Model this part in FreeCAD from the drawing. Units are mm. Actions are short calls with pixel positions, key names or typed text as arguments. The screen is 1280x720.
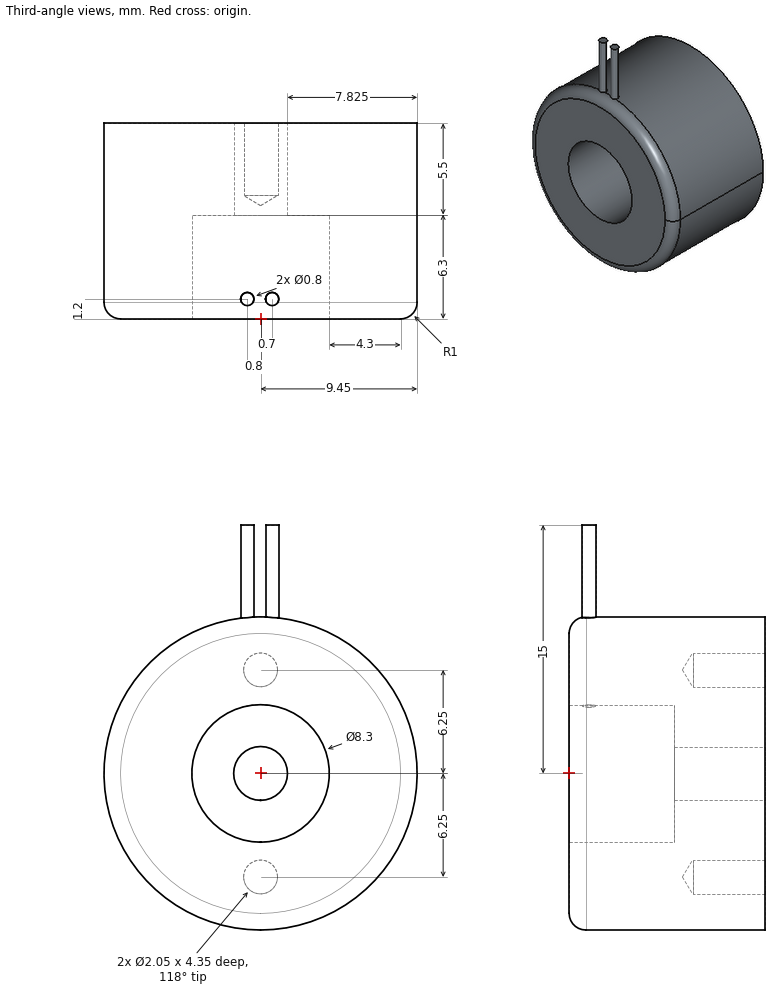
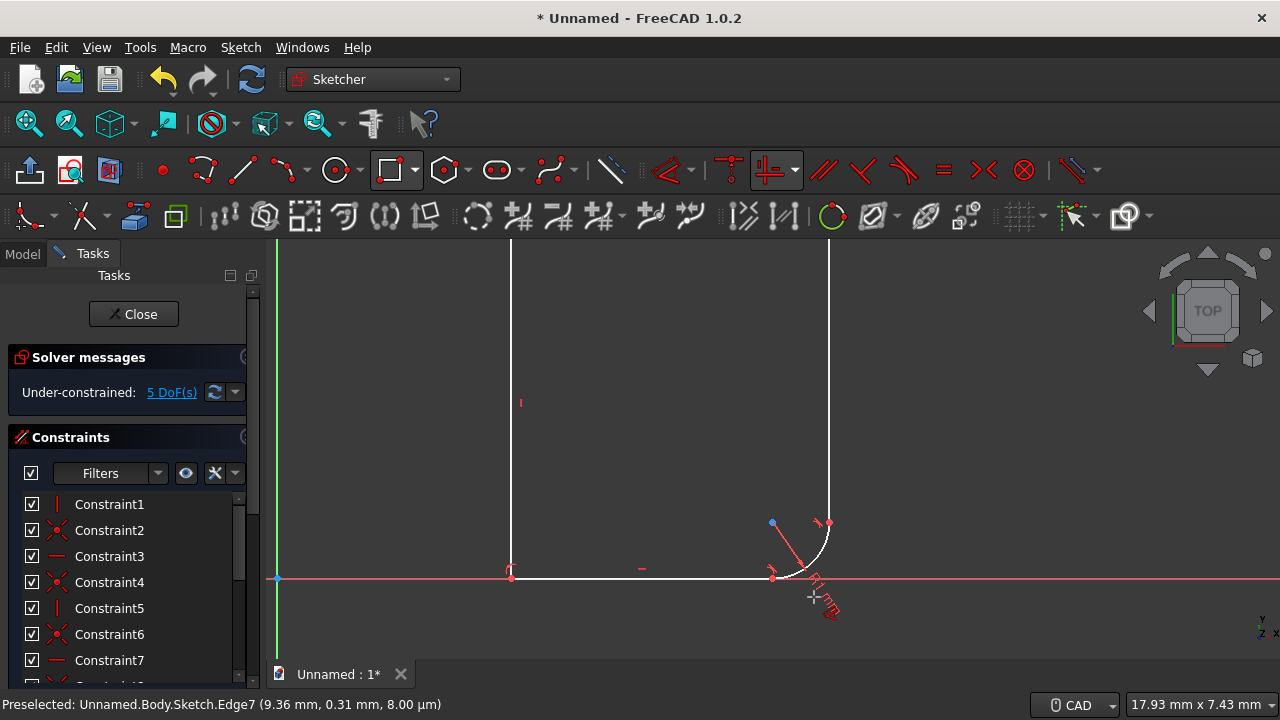
scroll(798, 568, down, 5)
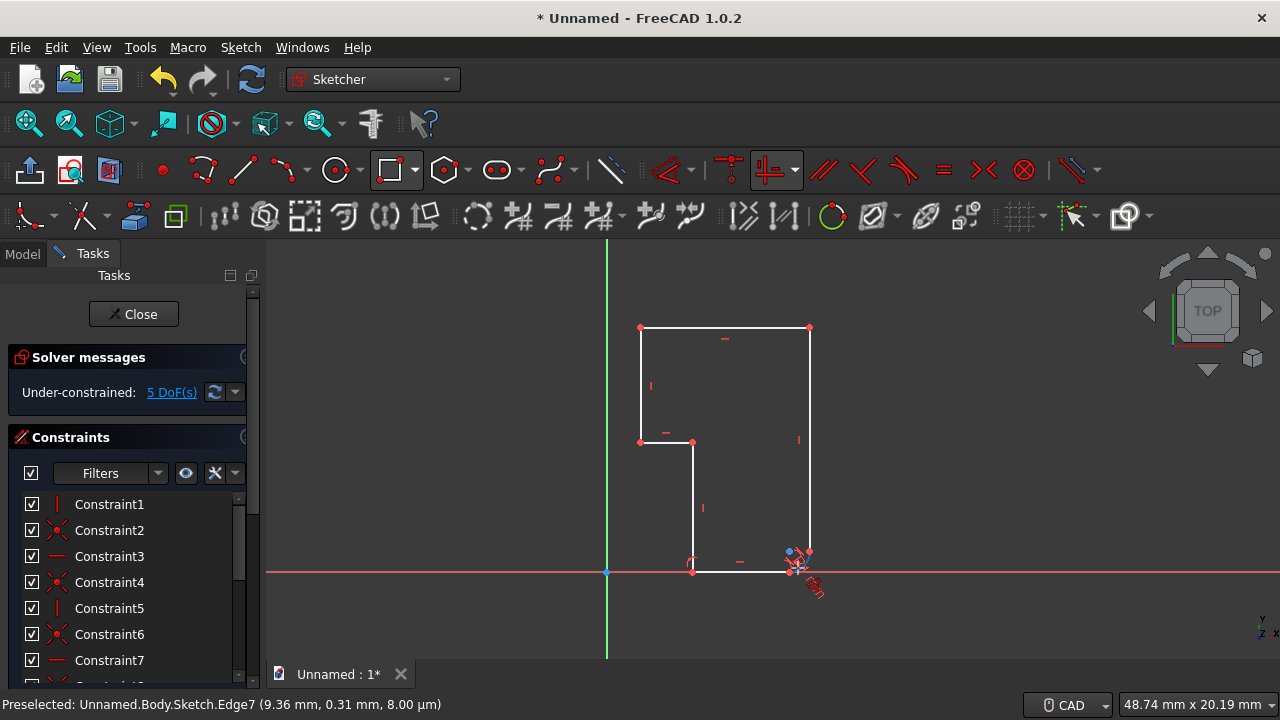
click(641, 362)
click(675, 385)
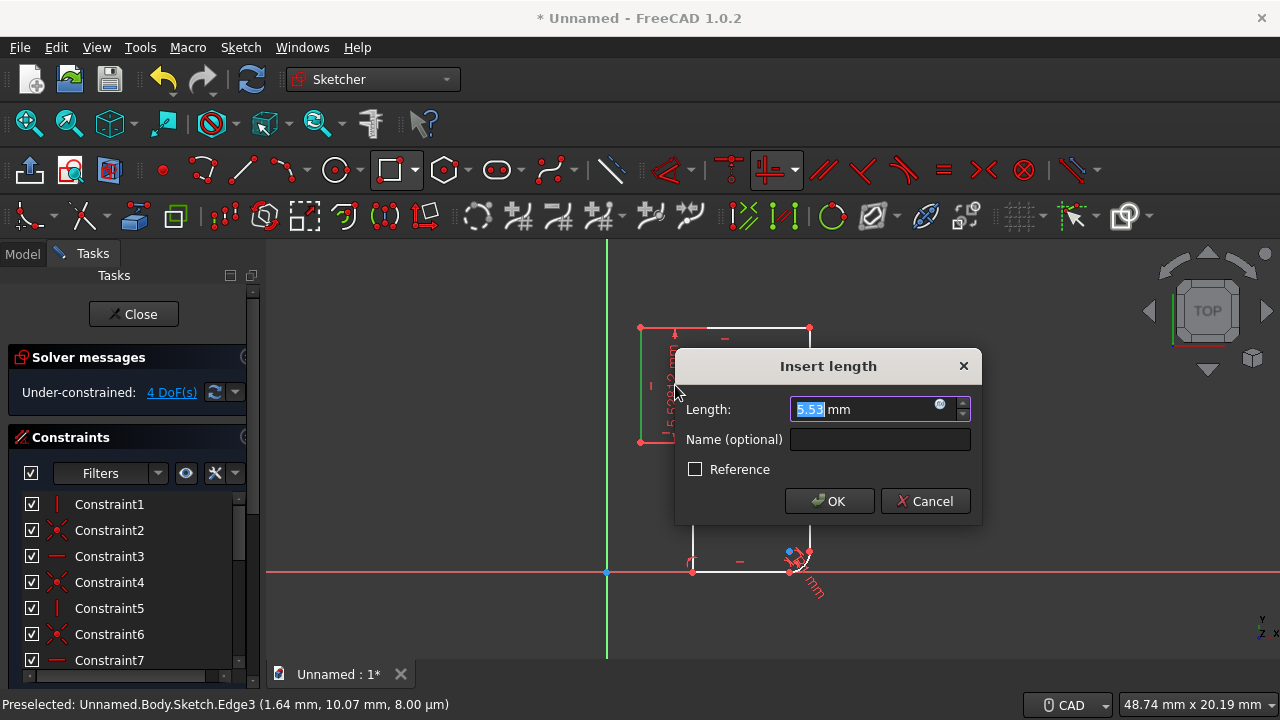
text(5.5)
key(Return)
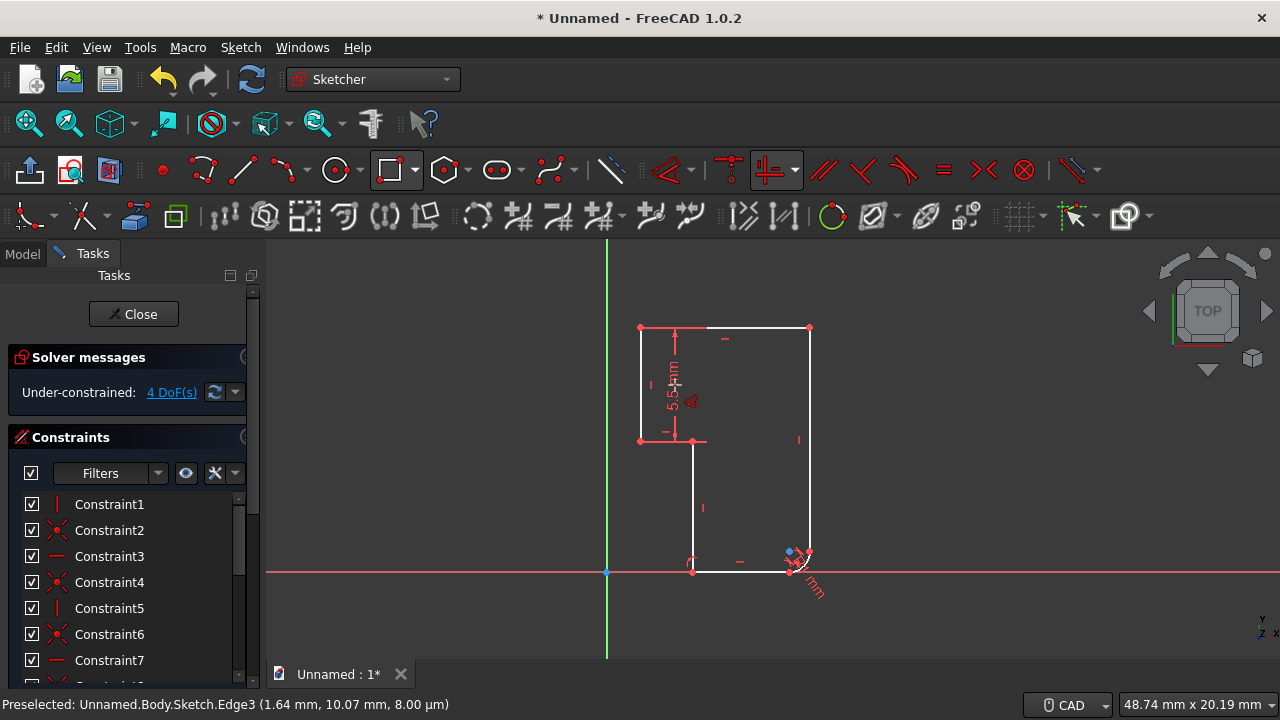
click(693, 481)
click(659, 507)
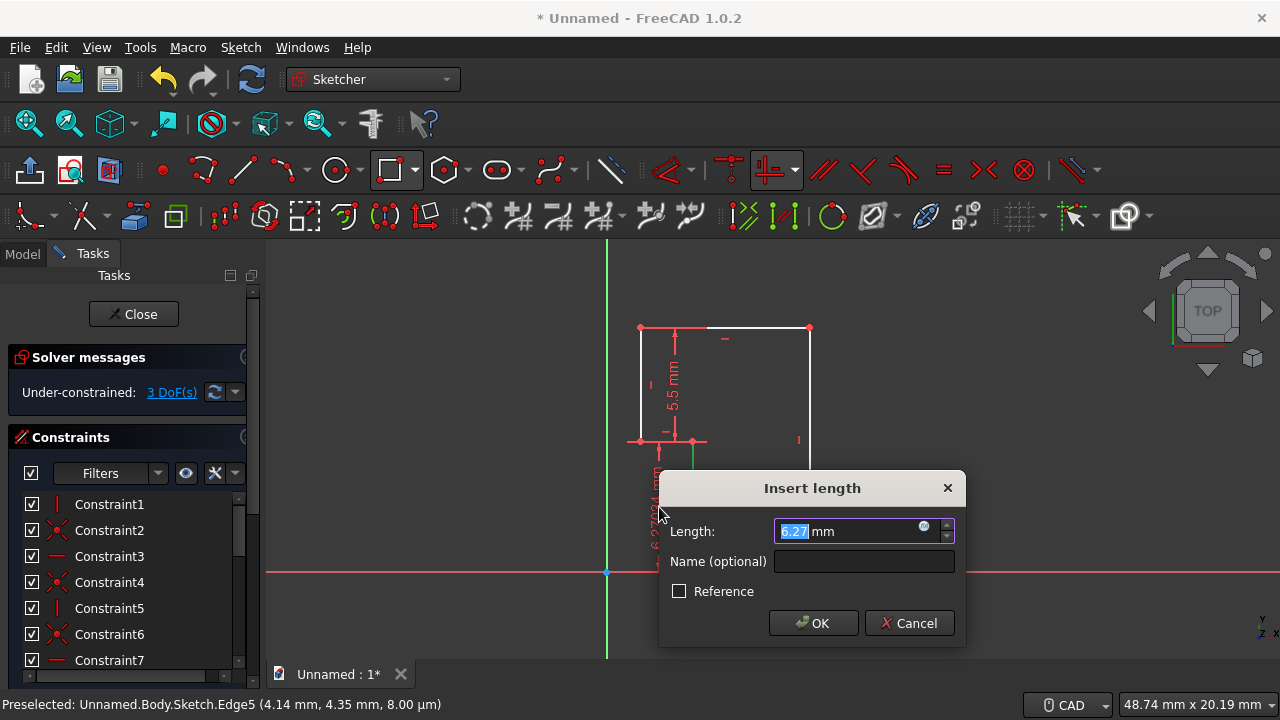
text(6.3)
key(Return)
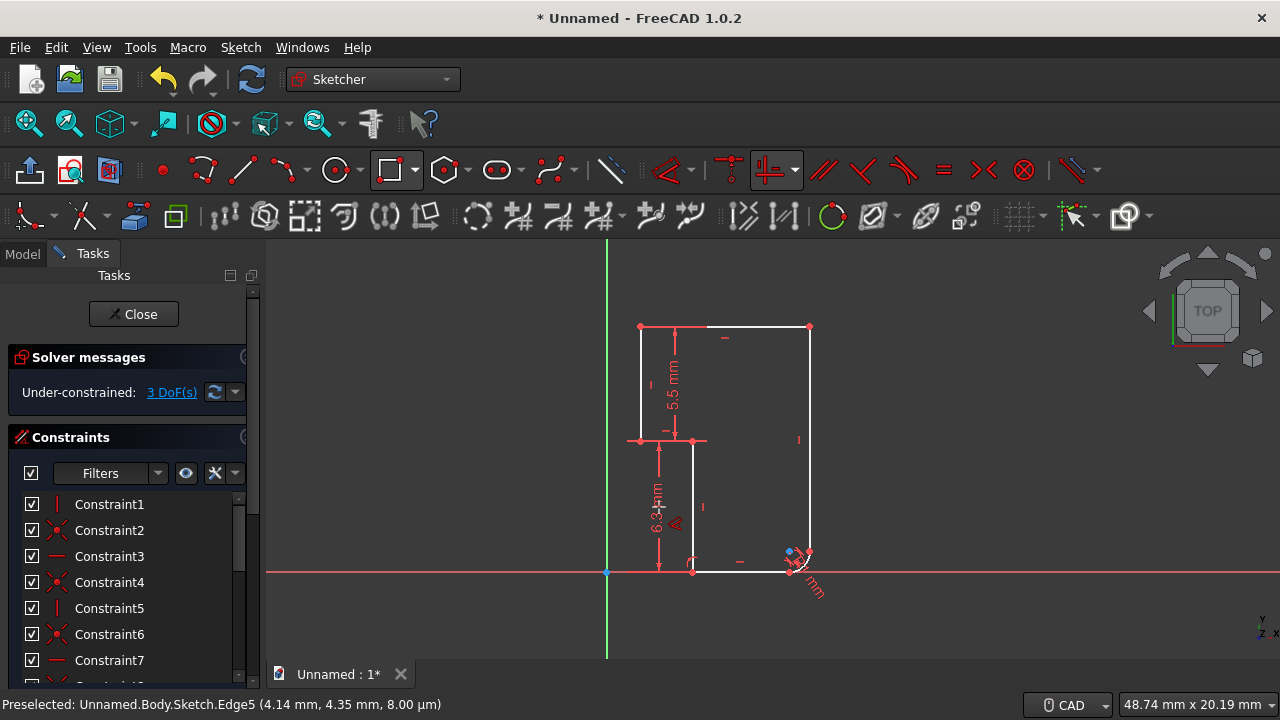
click(722, 572)
click(741, 606)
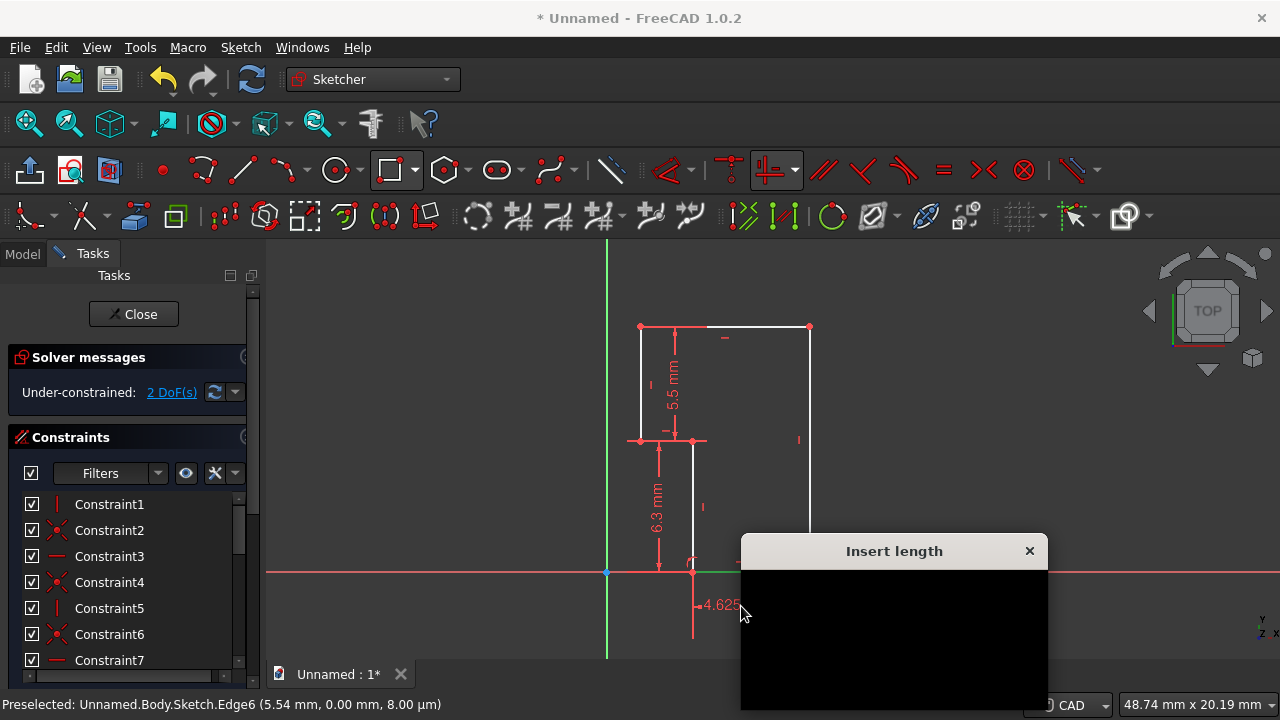
text(4.3)
key(Return)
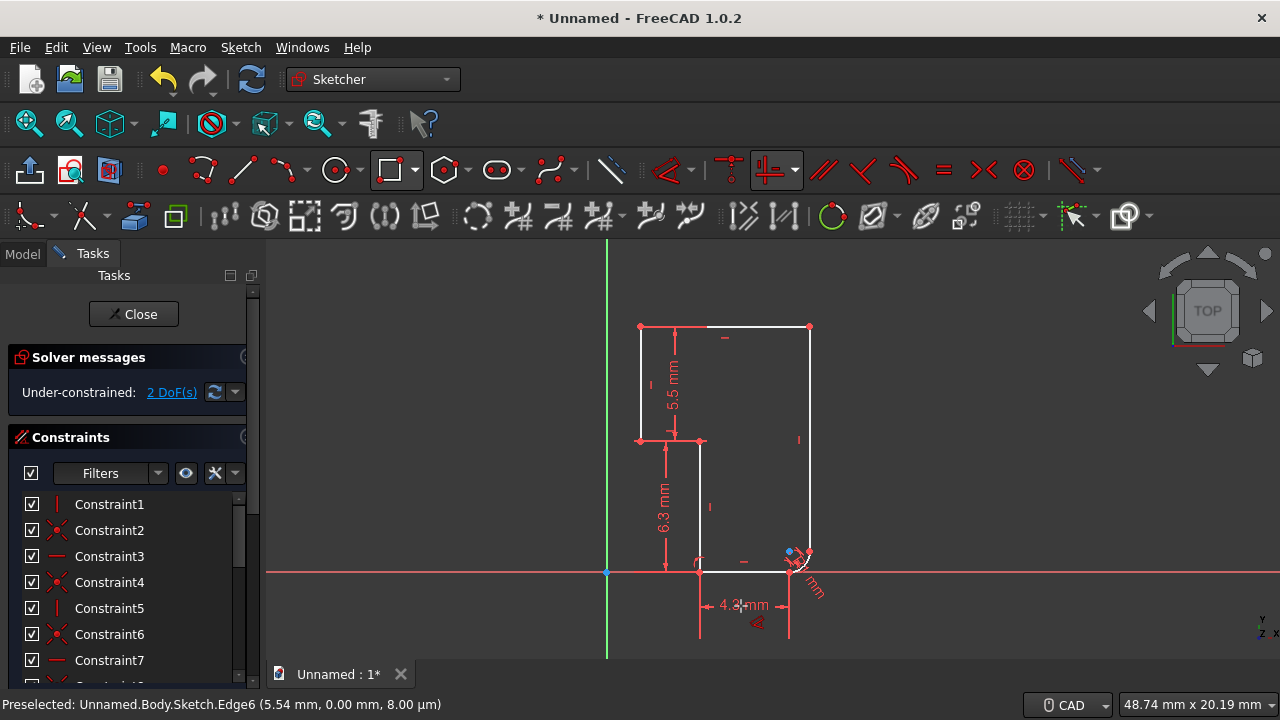
click(759, 327)
click(725, 293)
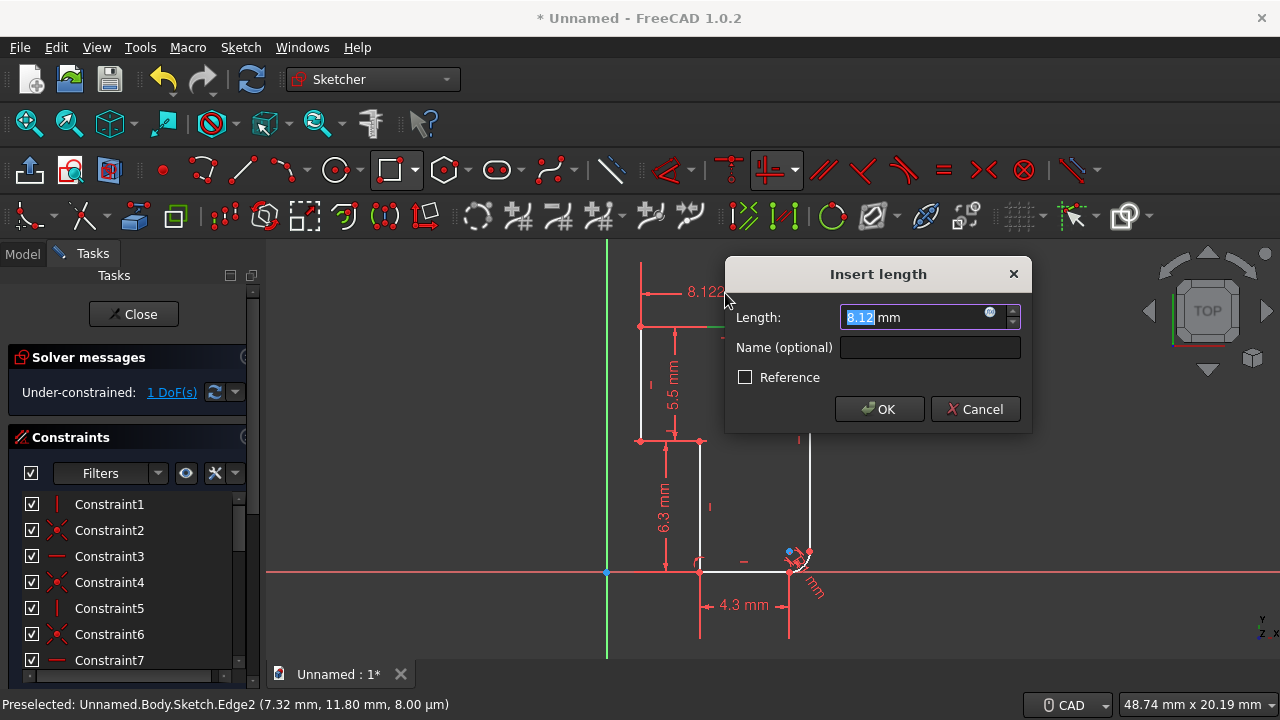
text(7.825)
key(Return)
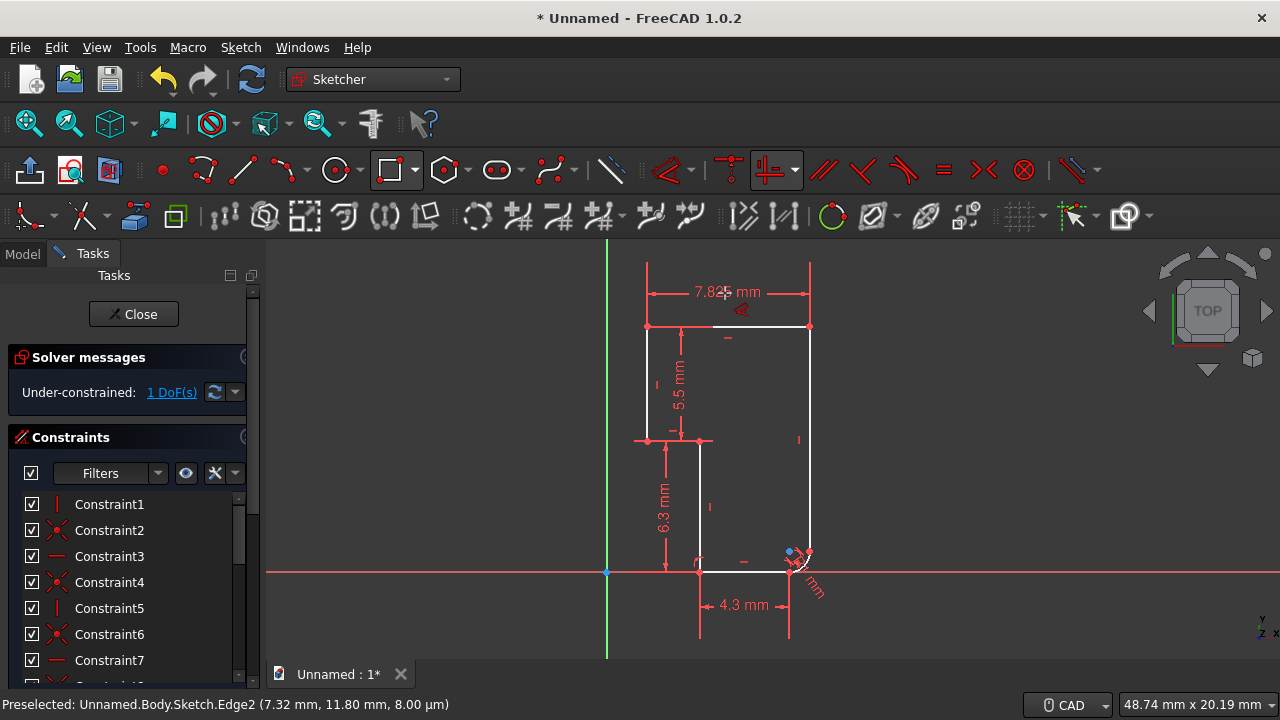
click(810, 552)
click(662, 606)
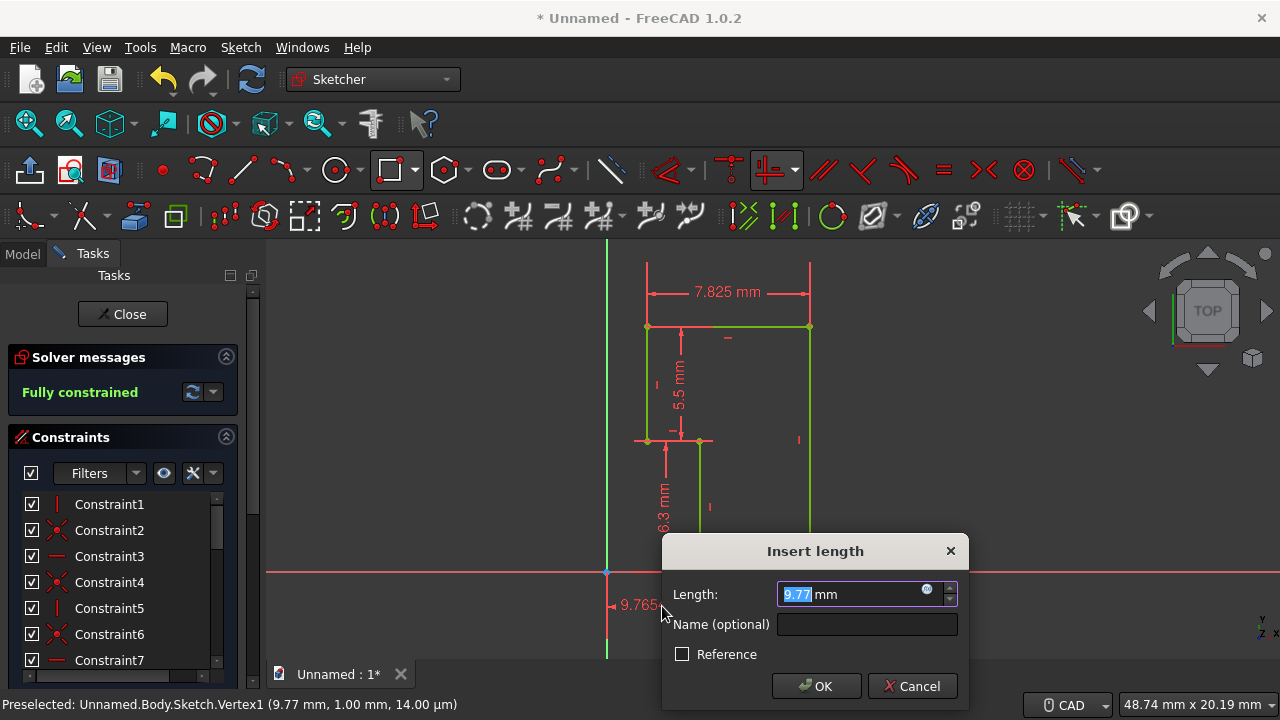
text(9.45)
key(Return)
key(Escape)